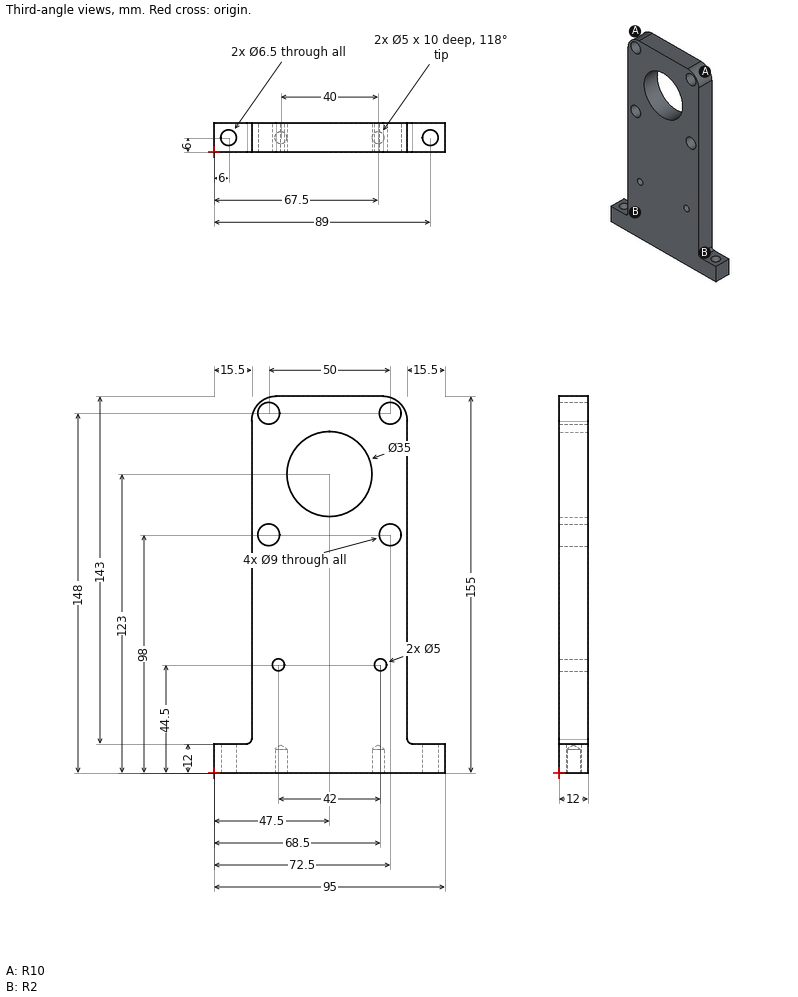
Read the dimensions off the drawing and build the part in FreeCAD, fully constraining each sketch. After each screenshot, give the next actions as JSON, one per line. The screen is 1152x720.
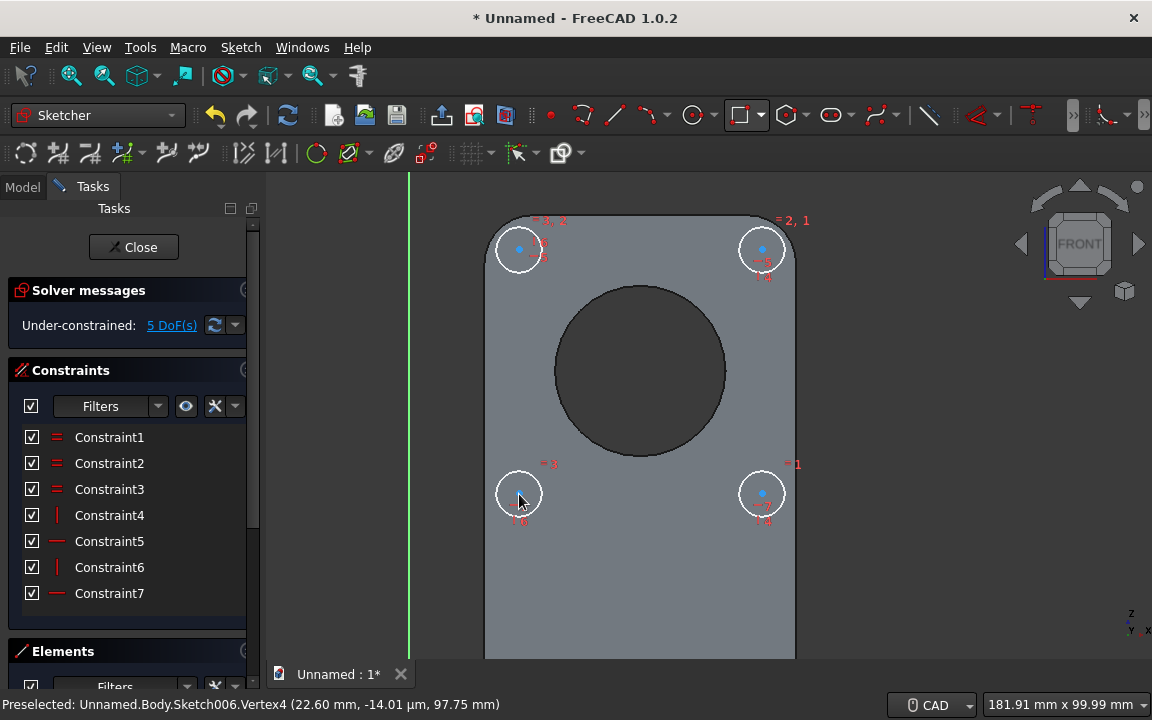
{"action": "left_click", "coordinate": [976, 116]}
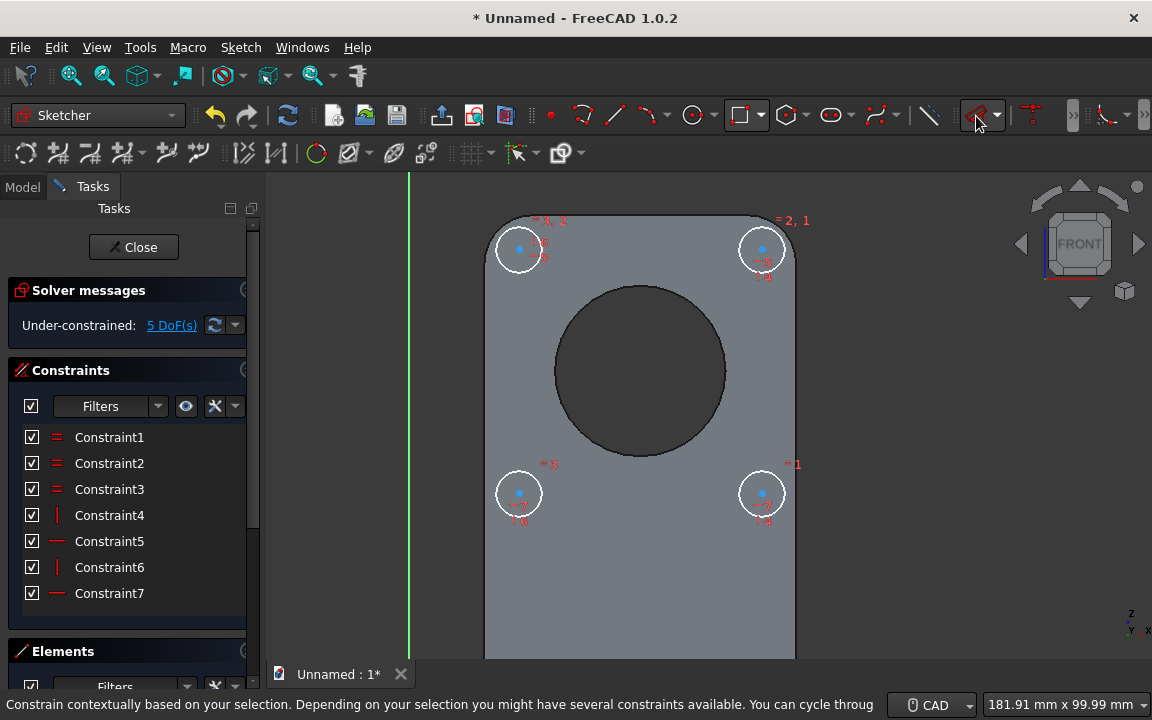
{"action": "left_click", "coordinate": [778, 478]}
{"action": "left_click", "coordinate": [801, 455]}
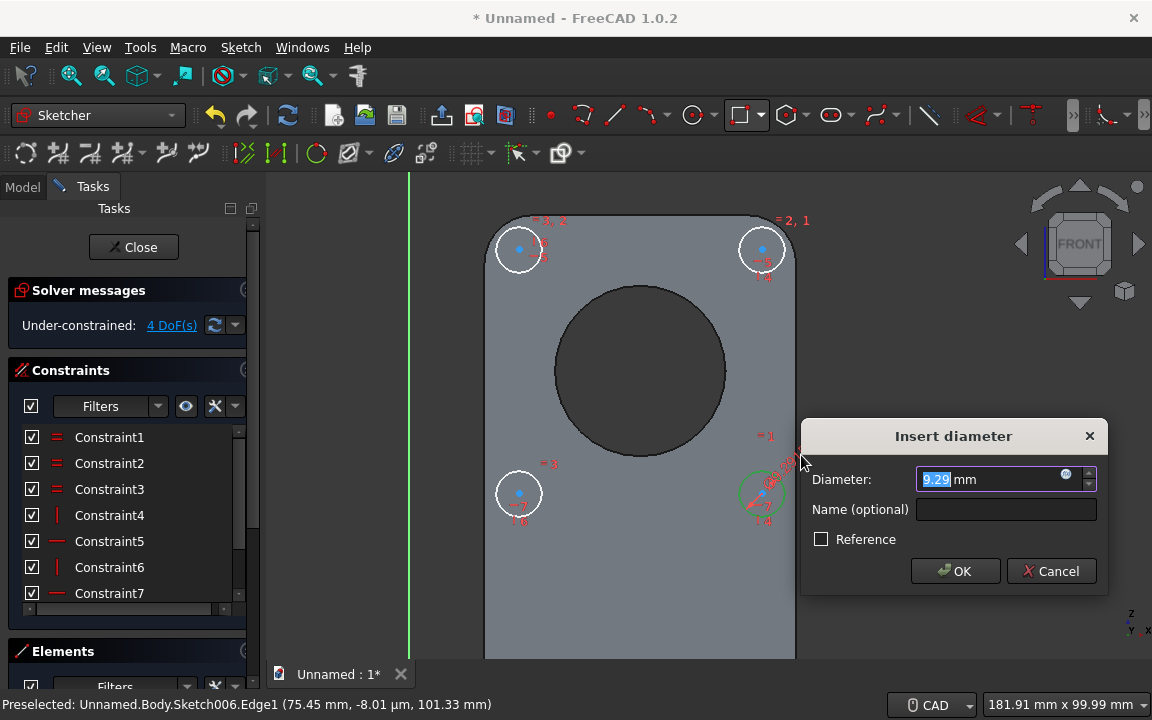
{"action": "type", "text": "9"}
{"action": "key", "text": "Return"}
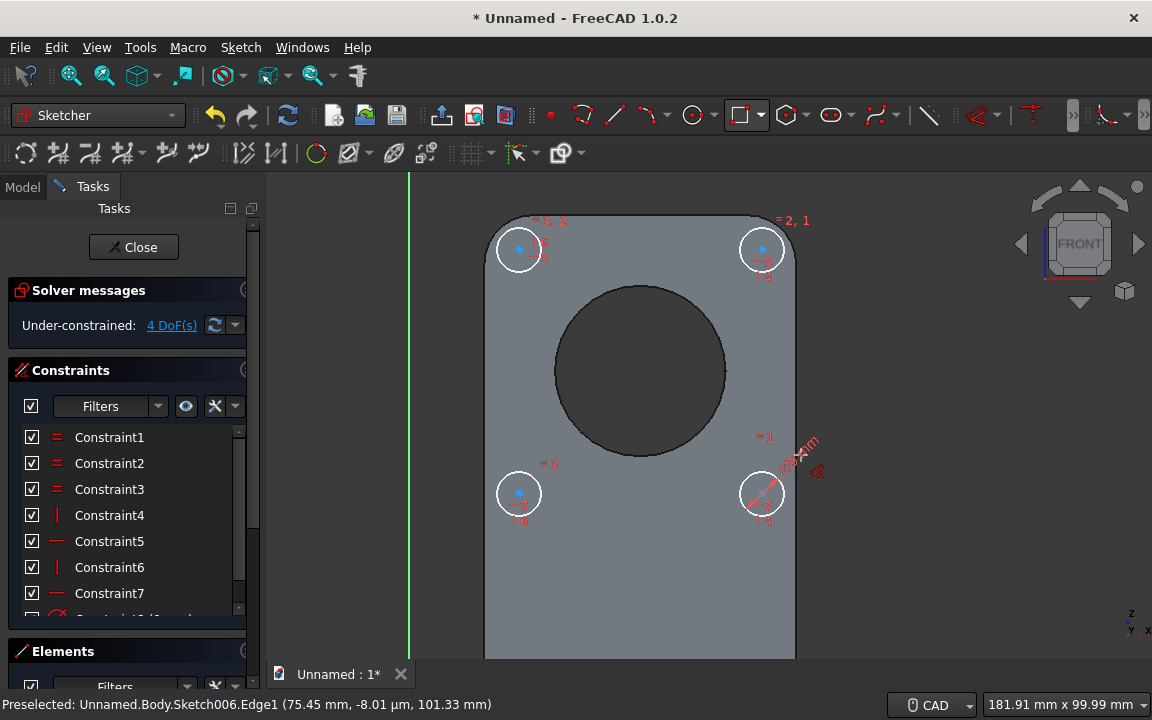
{"action": "left_click", "coordinate": [762, 494]}
{"action": "left_click", "coordinate": [375, 562]}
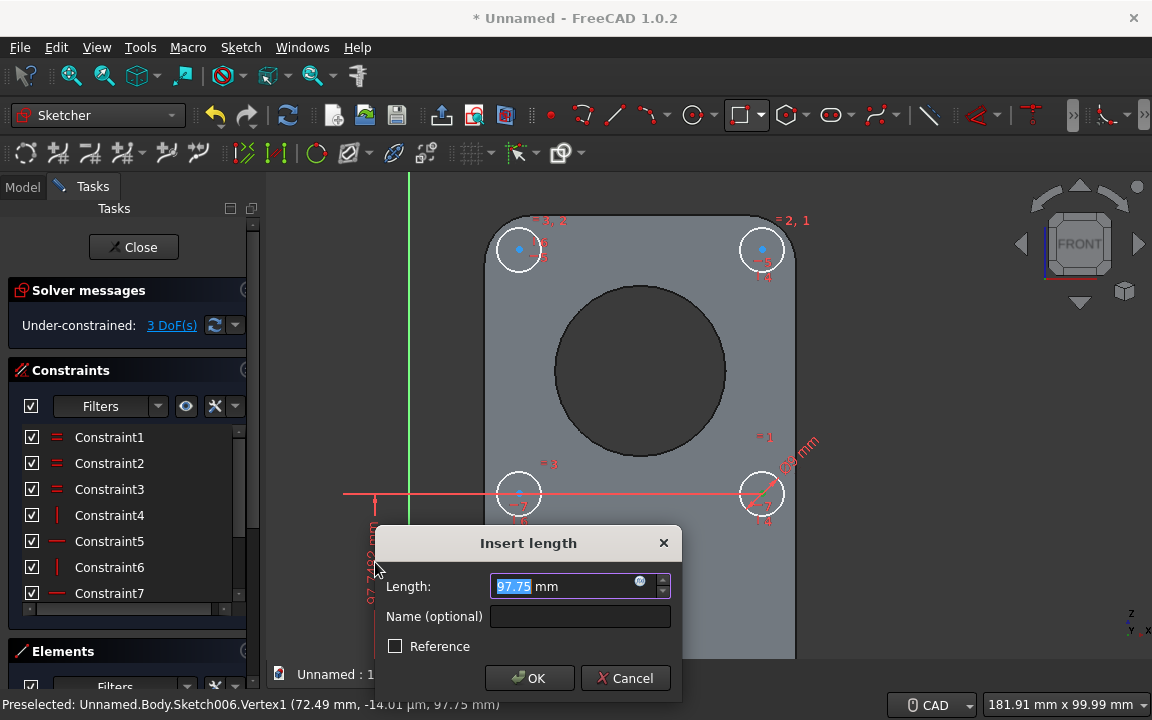
{"action": "type", "text": "98"}
{"action": "key", "text": "Return"}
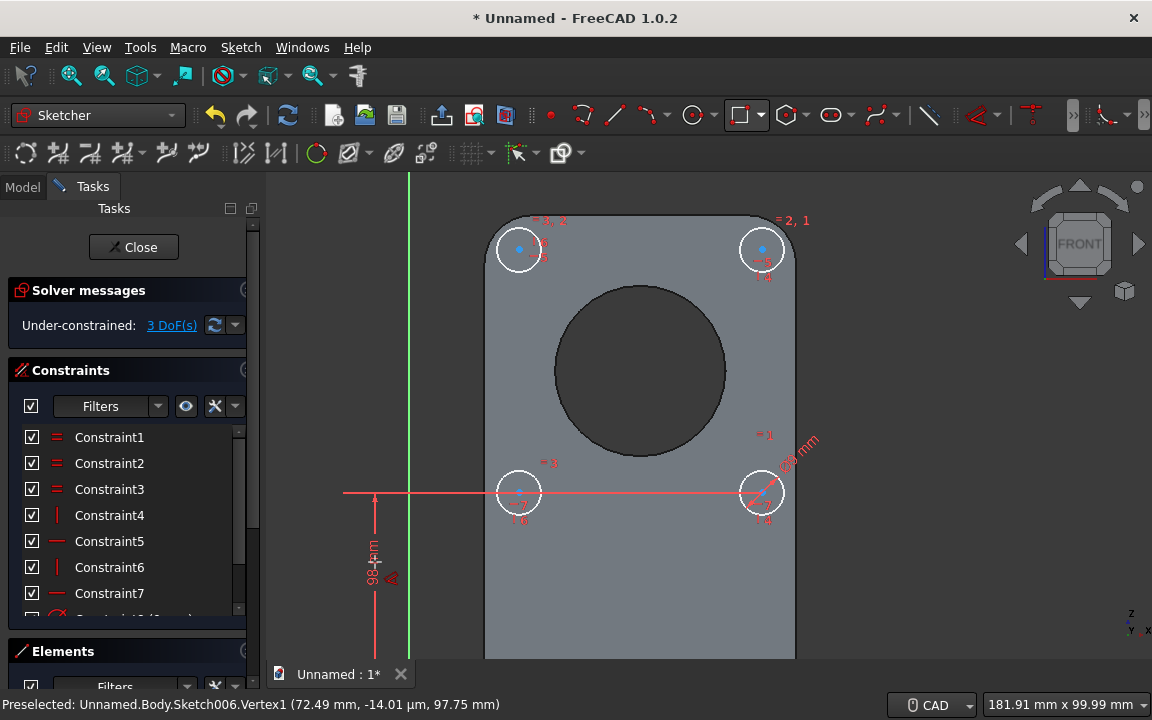
{"action": "left_click", "coordinate": [762, 250]}
{"action": "left_click", "coordinate": [375, 441]}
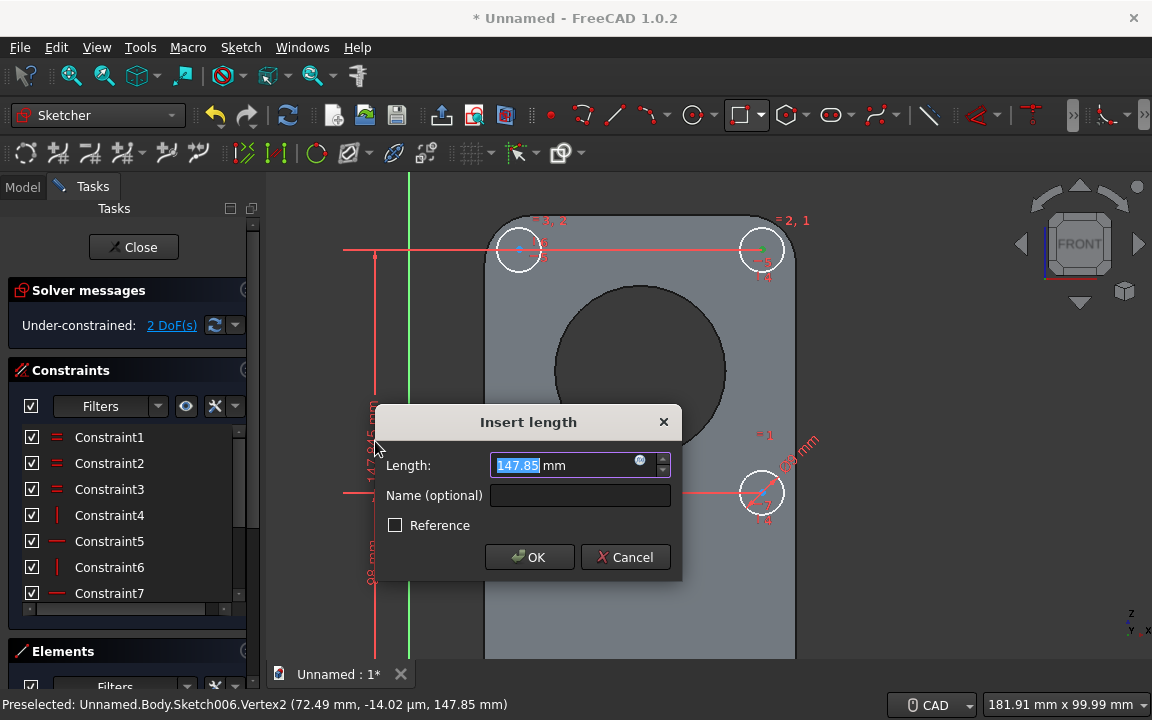
{"action": "type", "text": "148"}
{"action": "key", "text": "Return"}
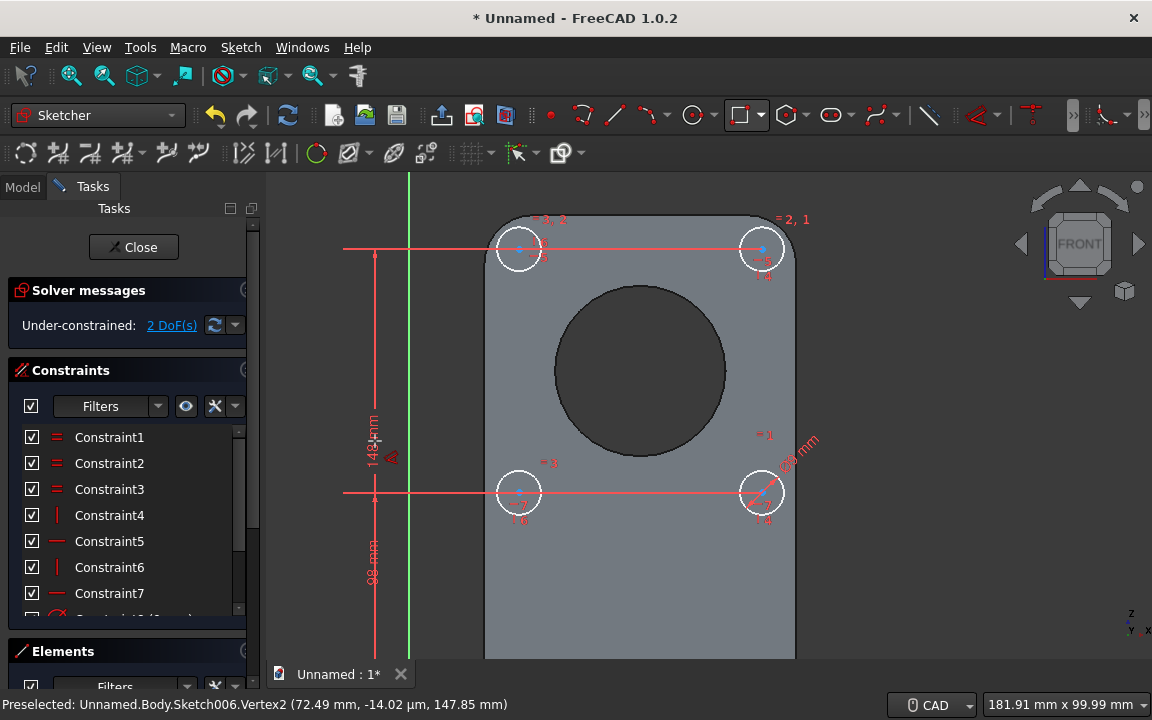
{"action": "left_click", "coordinate": [762, 249]}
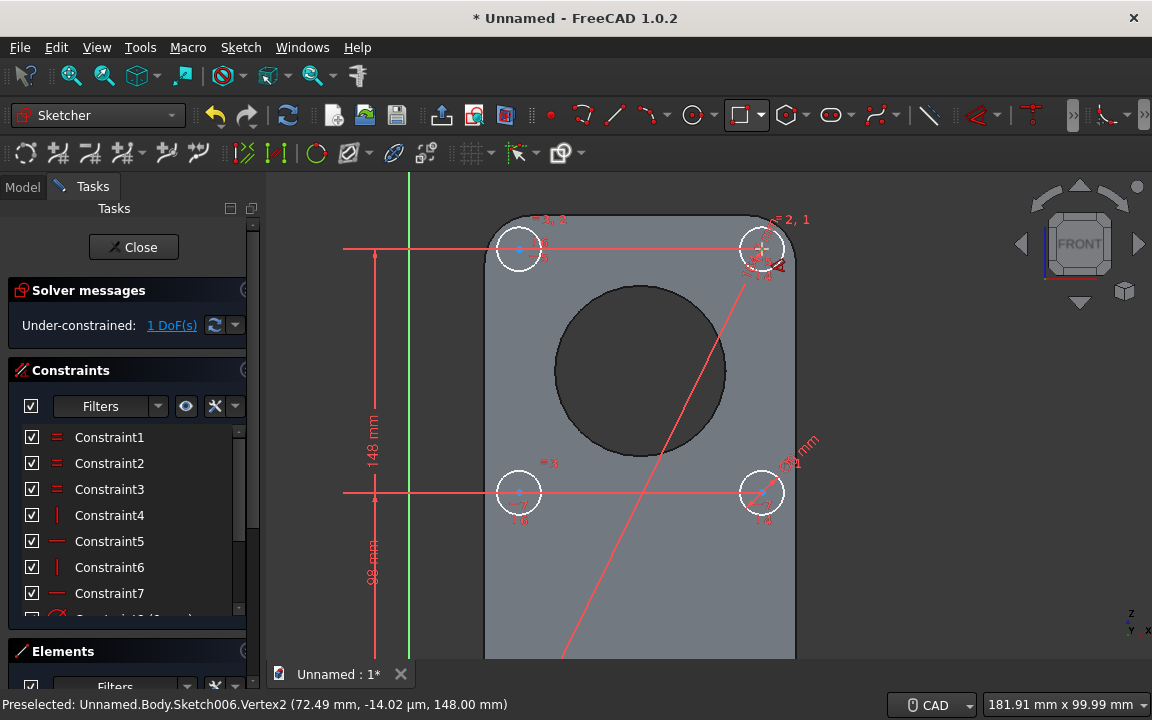
{"action": "left_click", "coordinate": [519, 249]}
{"action": "left_click", "coordinate": [640, 215]}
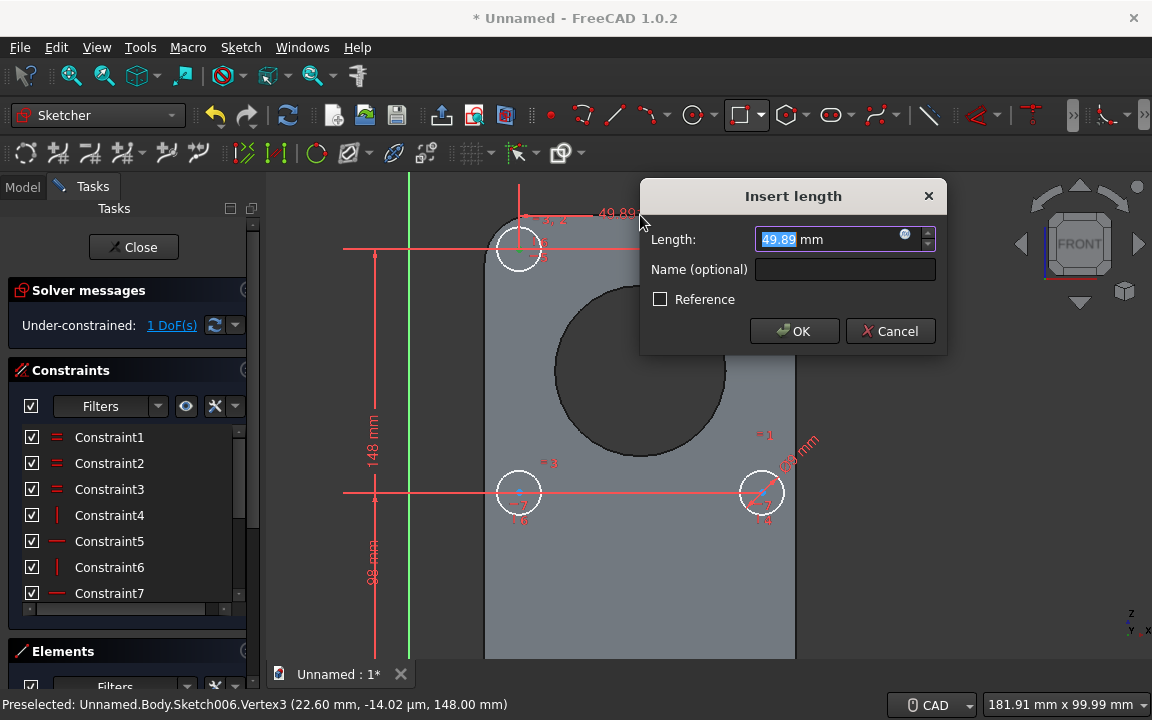
{"action": "type", "text": "50"}
{"action": "key", "text": "Return"}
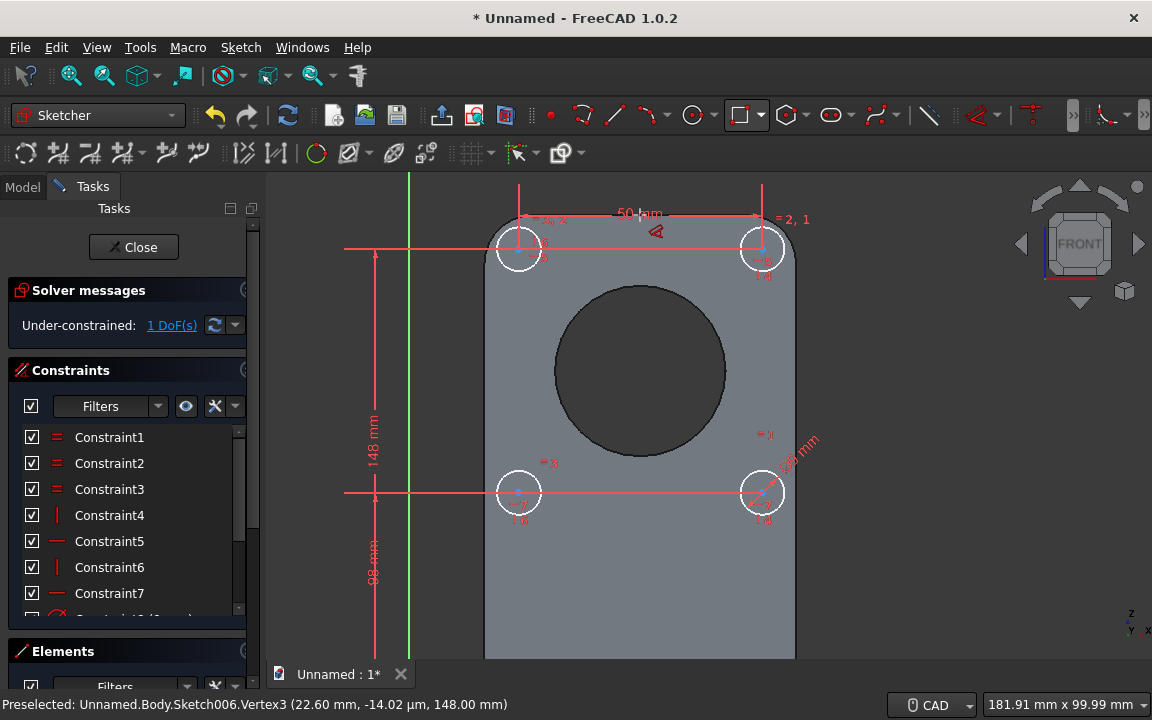
{"action": "left_click", "coordinate": [762, 493]}
{"action": "left_click", "coordinate": [586, 459]}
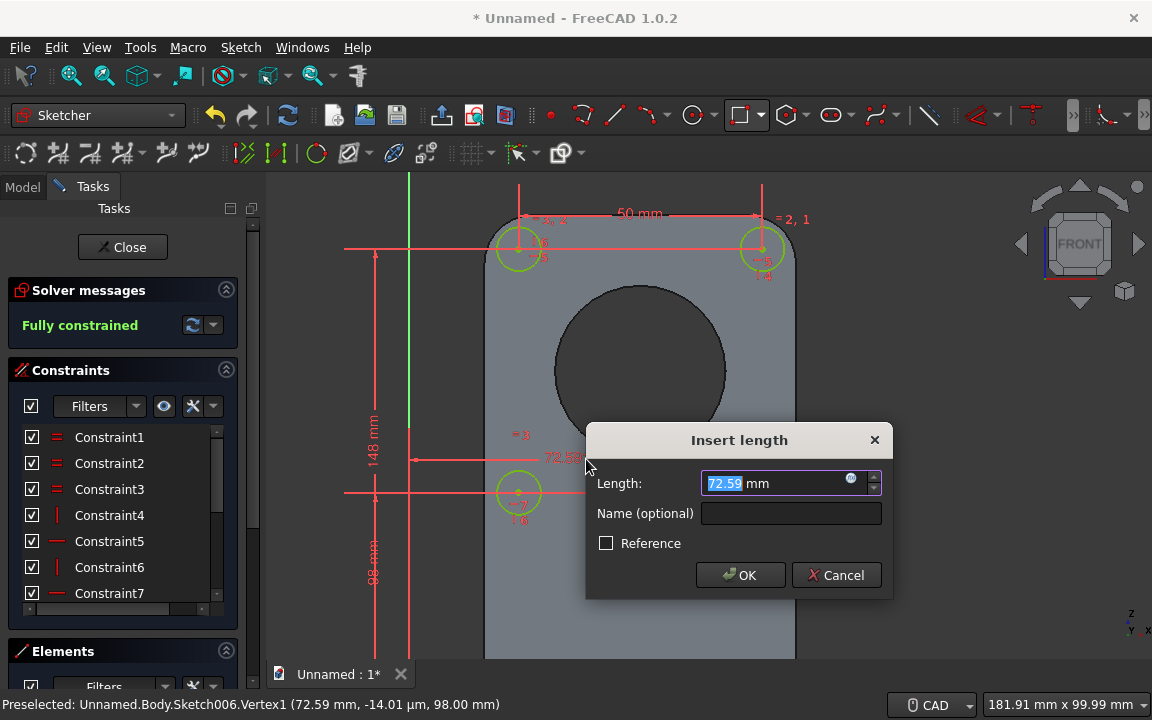
{"action": "type", "text": "72.5"}
{"action": "key", "text": "Return"}
{"action": "key", "text": "Escape"}